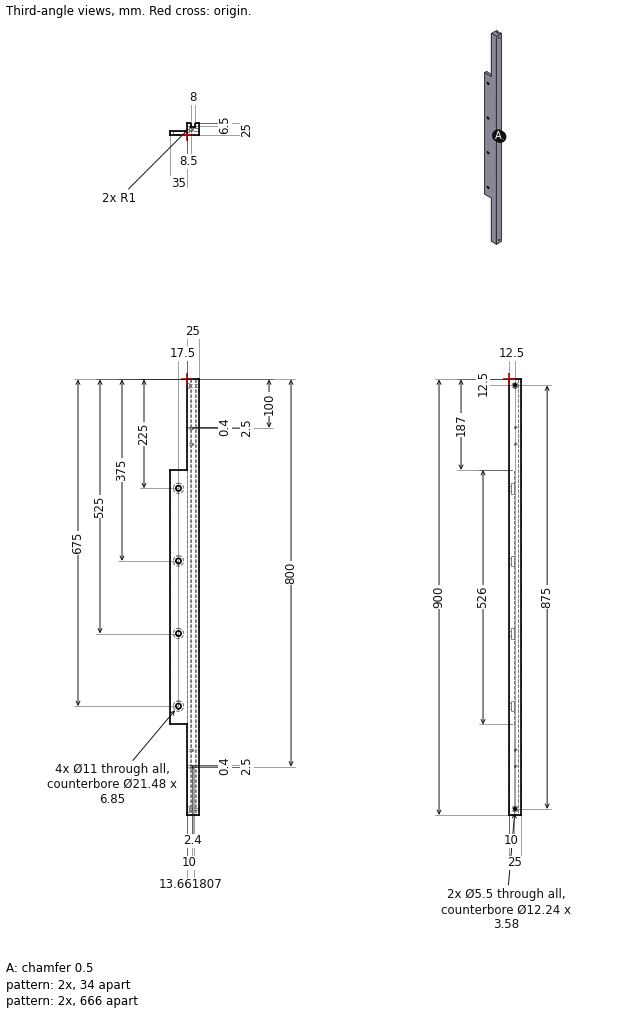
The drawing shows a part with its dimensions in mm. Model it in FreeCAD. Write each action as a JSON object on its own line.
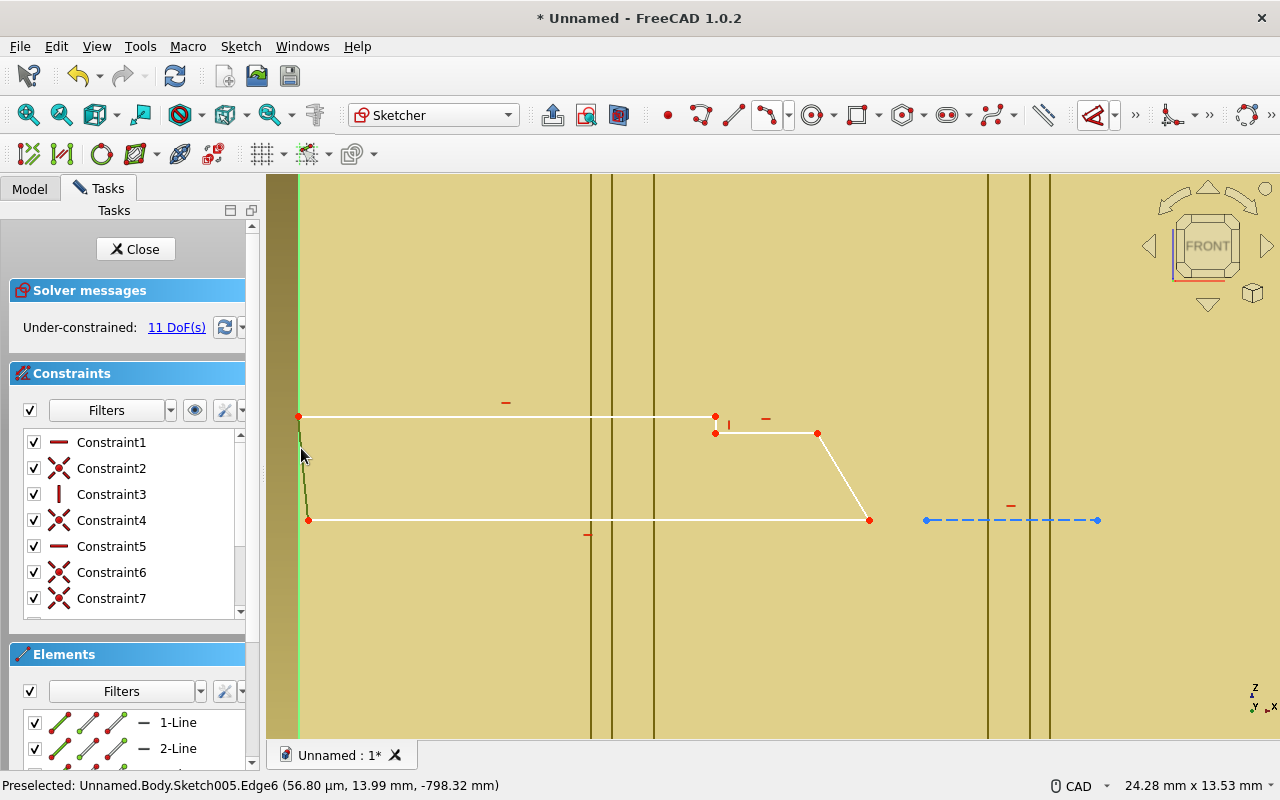
{"action": "key", "text": "v"}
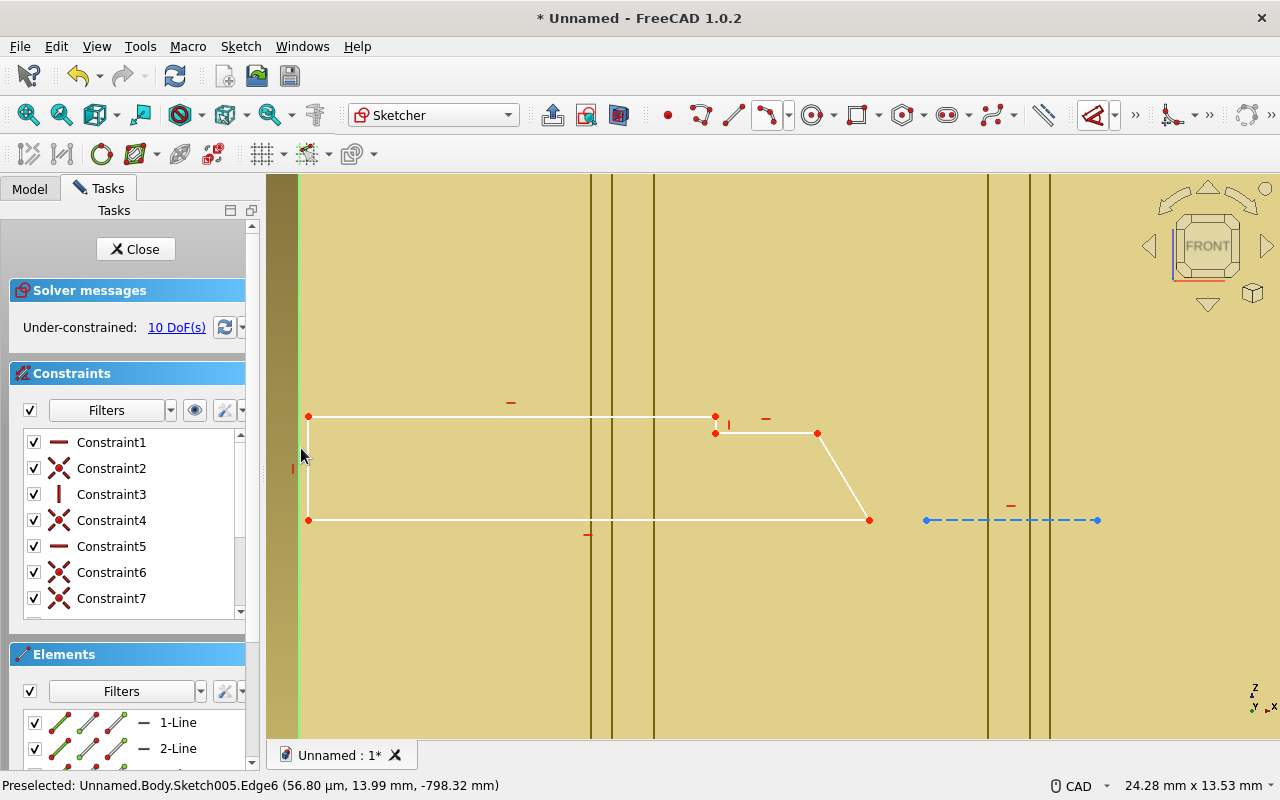
{"action": "left_click", "coordinate": [308, 417]}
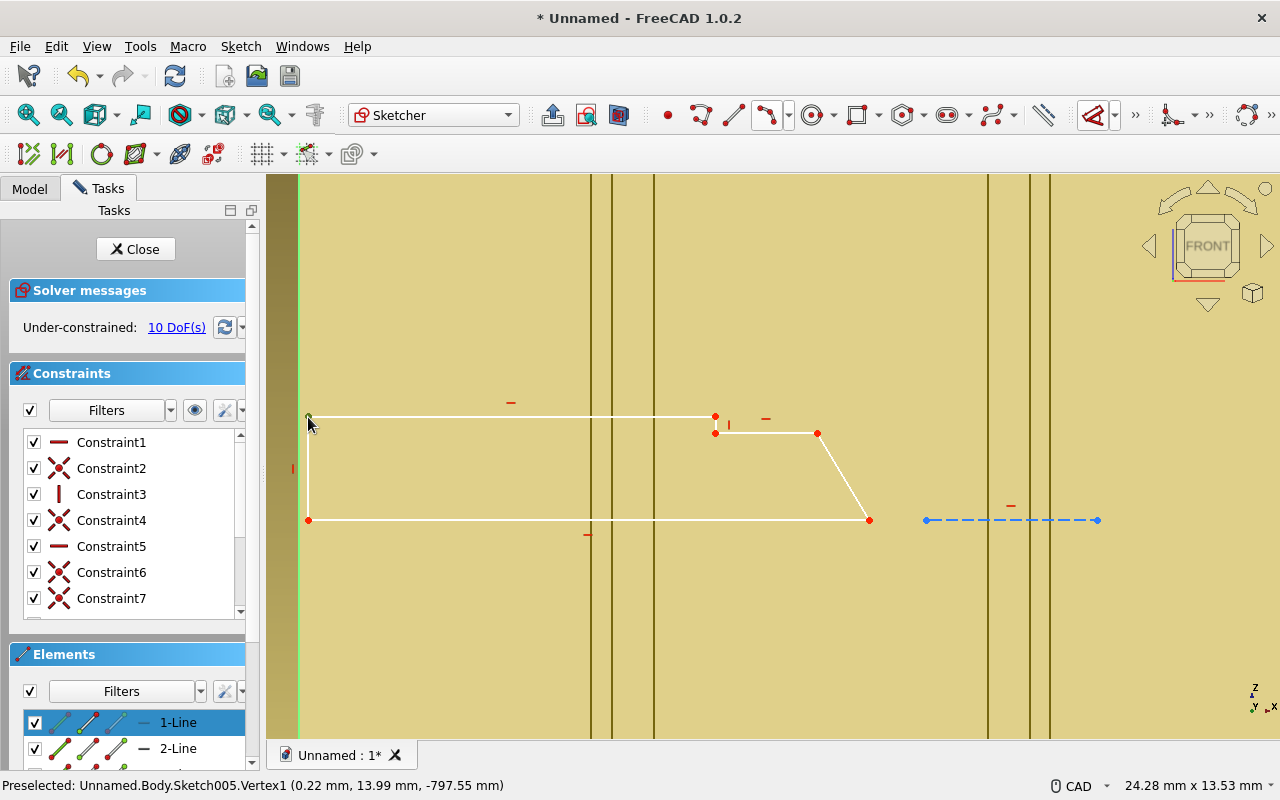
{"action": "left_click", "coordinate": [299, 675]}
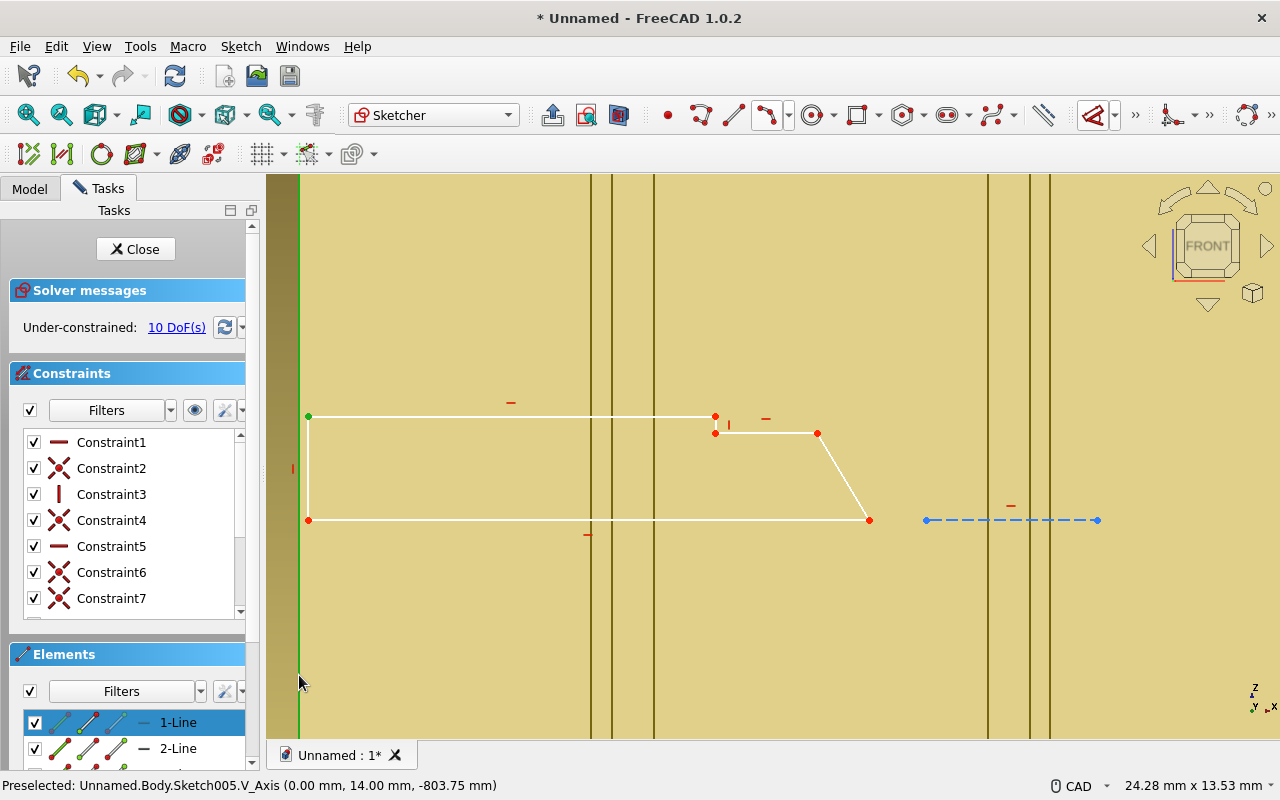
{"action": "key", "text": "c"}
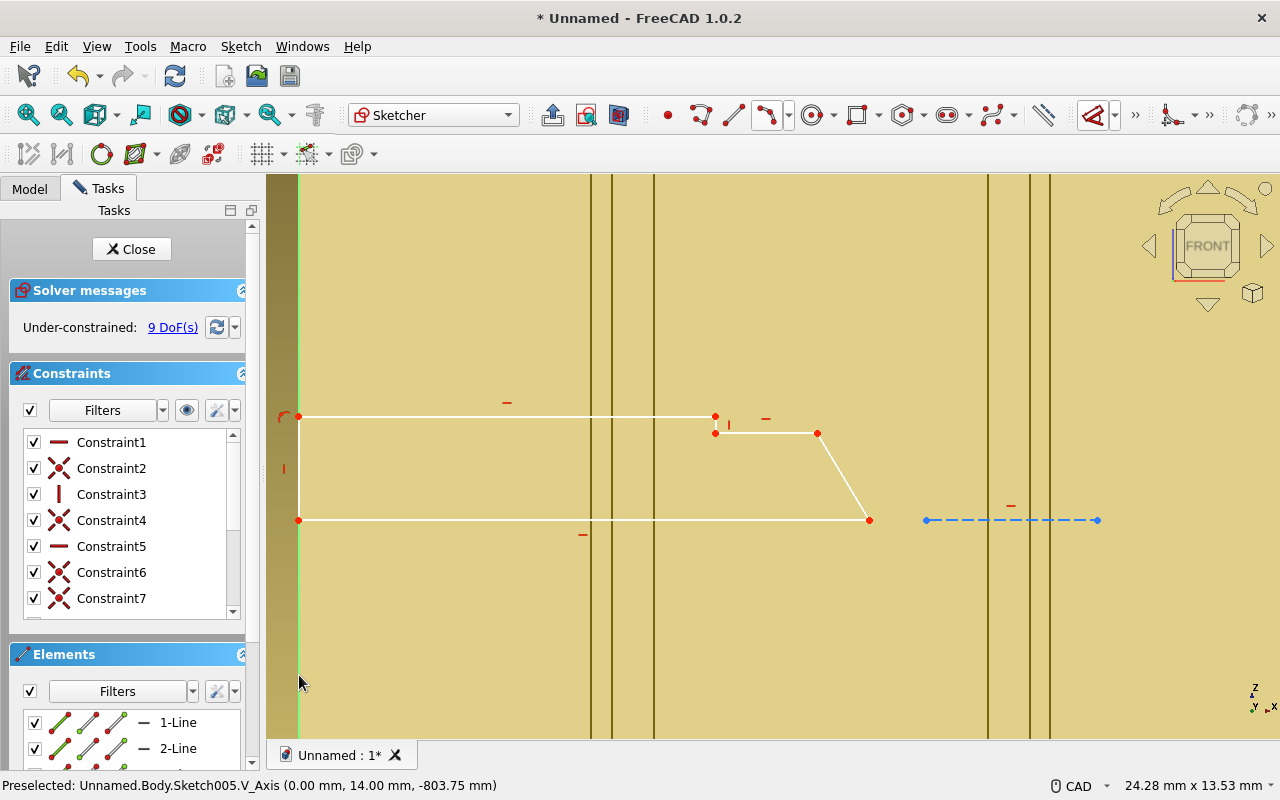
{"action": "left_click", "coordinate": [424, 417]}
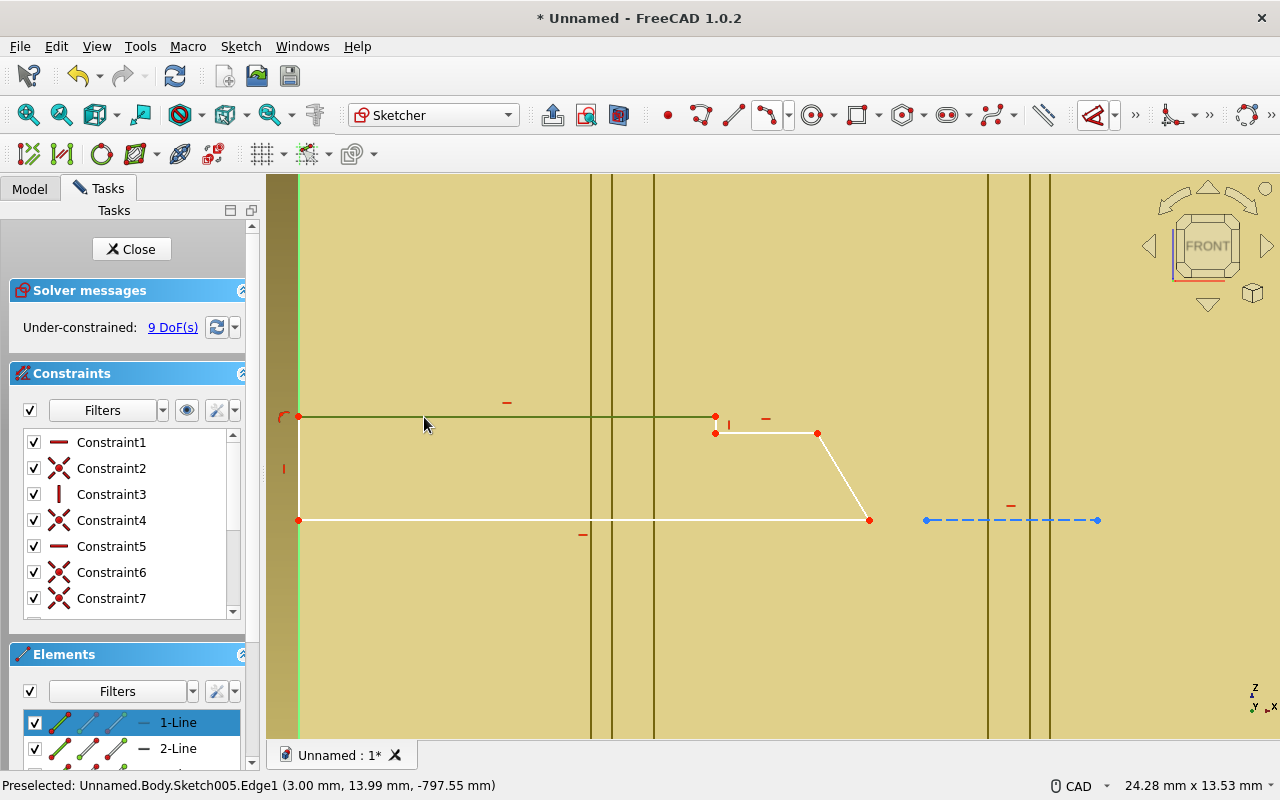
{"action": "left_click", "coordinate": [1114, 116]}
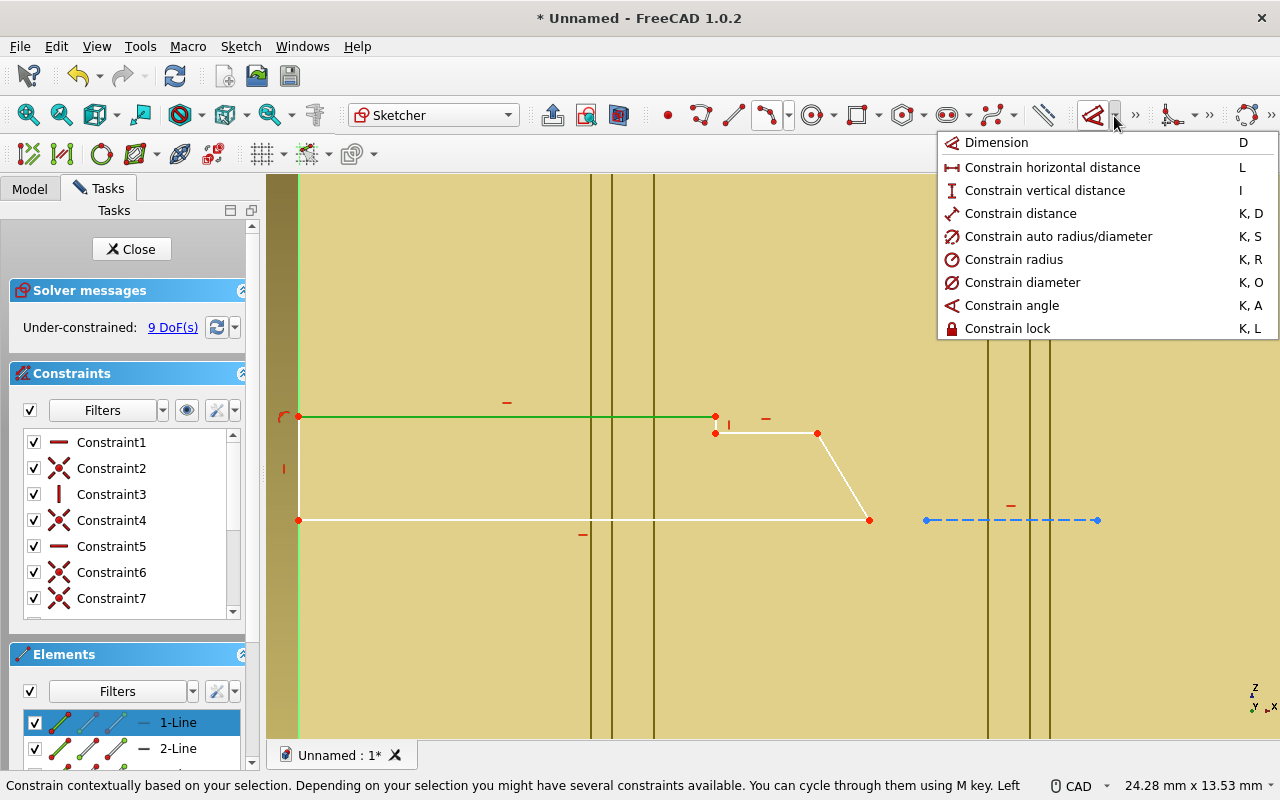
{"action": "left_click", "coordinate": [1108, 168]}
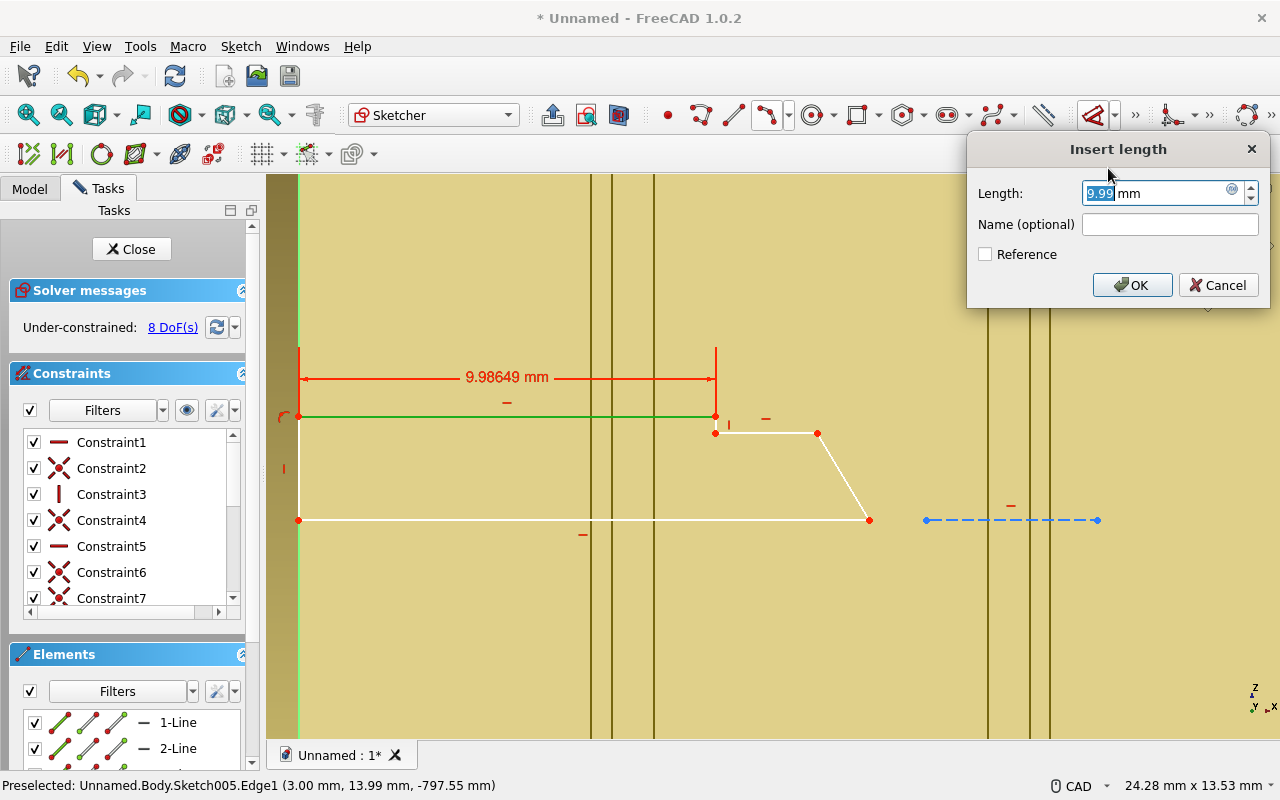
{"action": "type", "text": "10"}
{"action": "key", "text": "Return"}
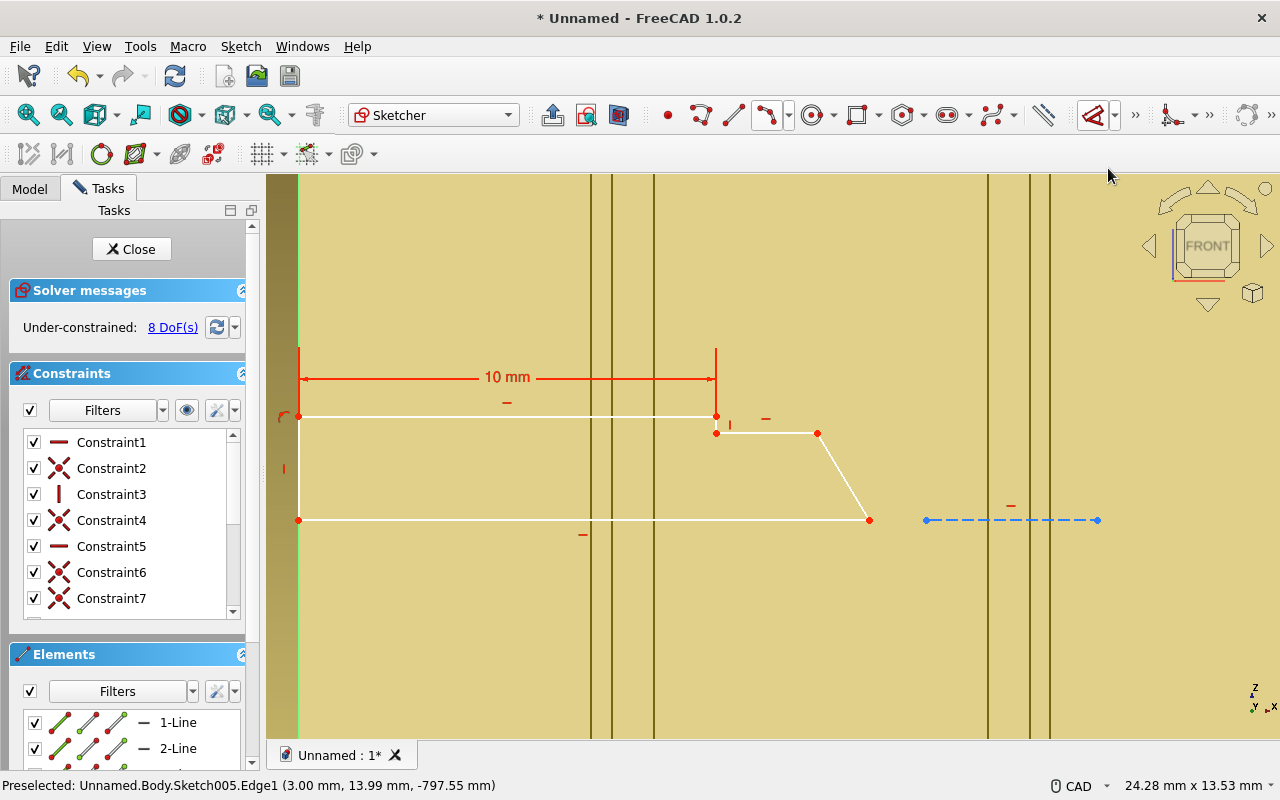
{"action": "scroll", "coordinate": [716, 425], "scroll_direction": "up", "scroll_amount": 5}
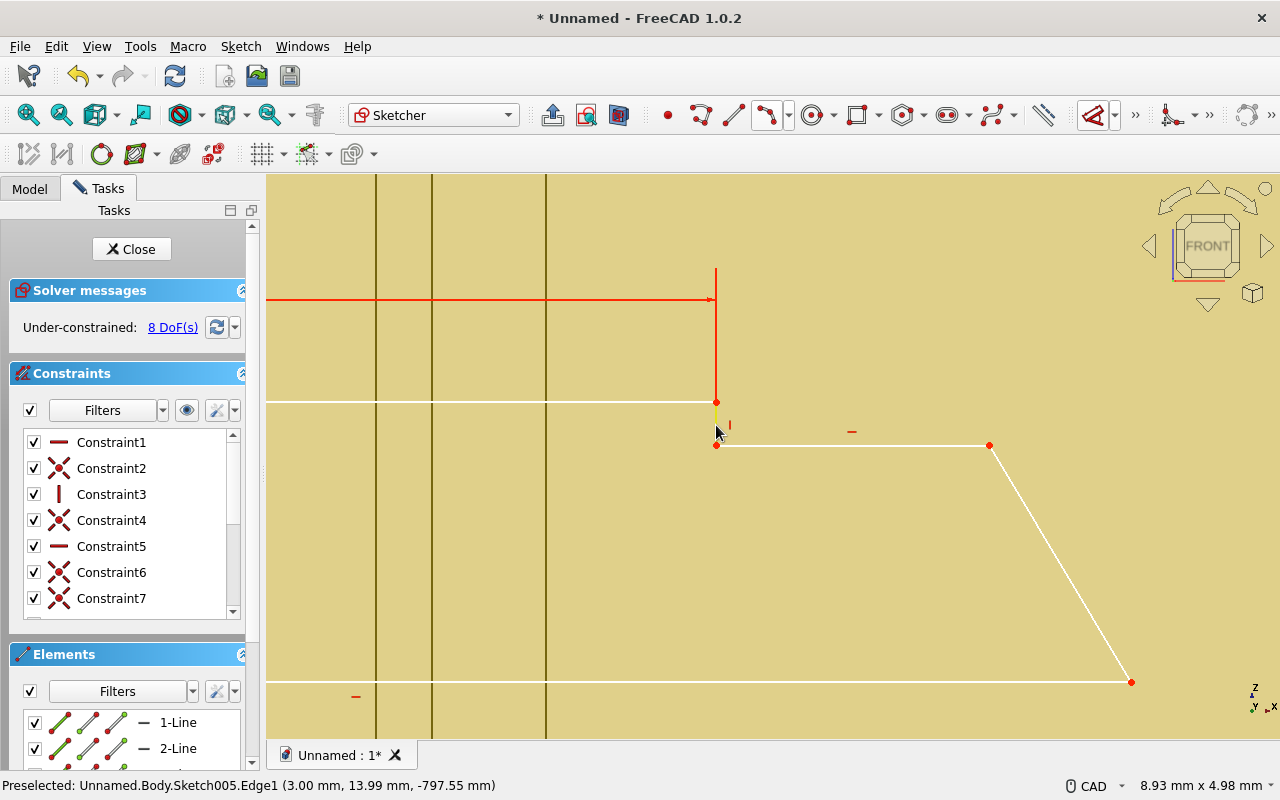
{"action": "left_click", "coordinate": [716, 424]}